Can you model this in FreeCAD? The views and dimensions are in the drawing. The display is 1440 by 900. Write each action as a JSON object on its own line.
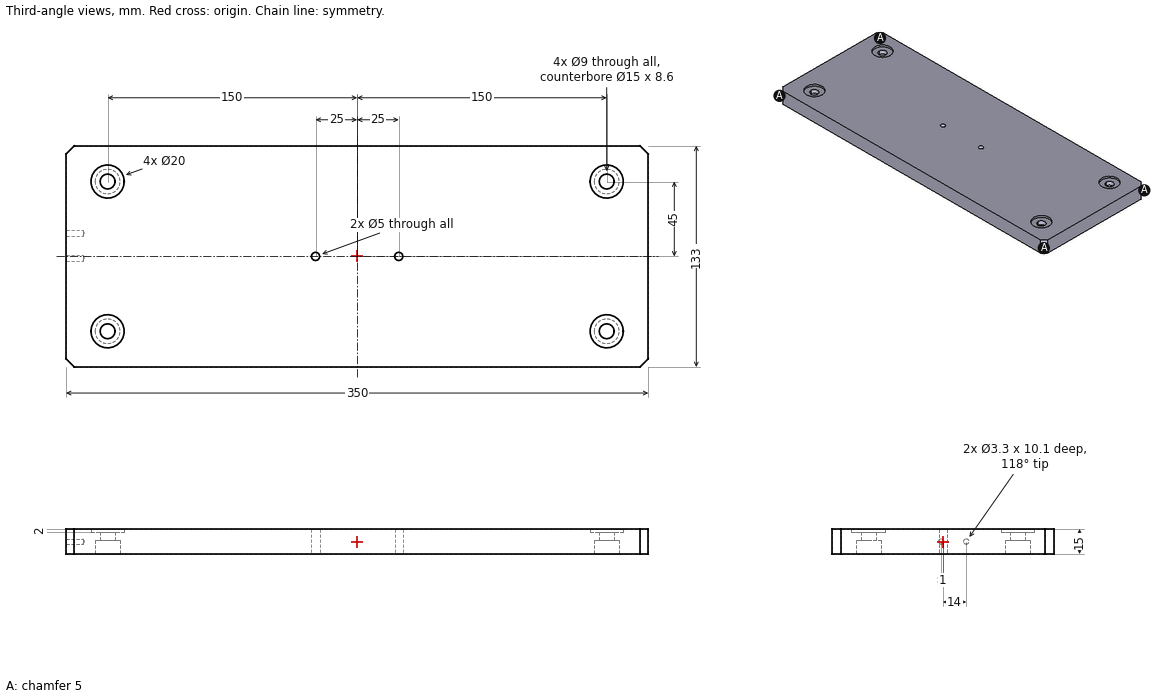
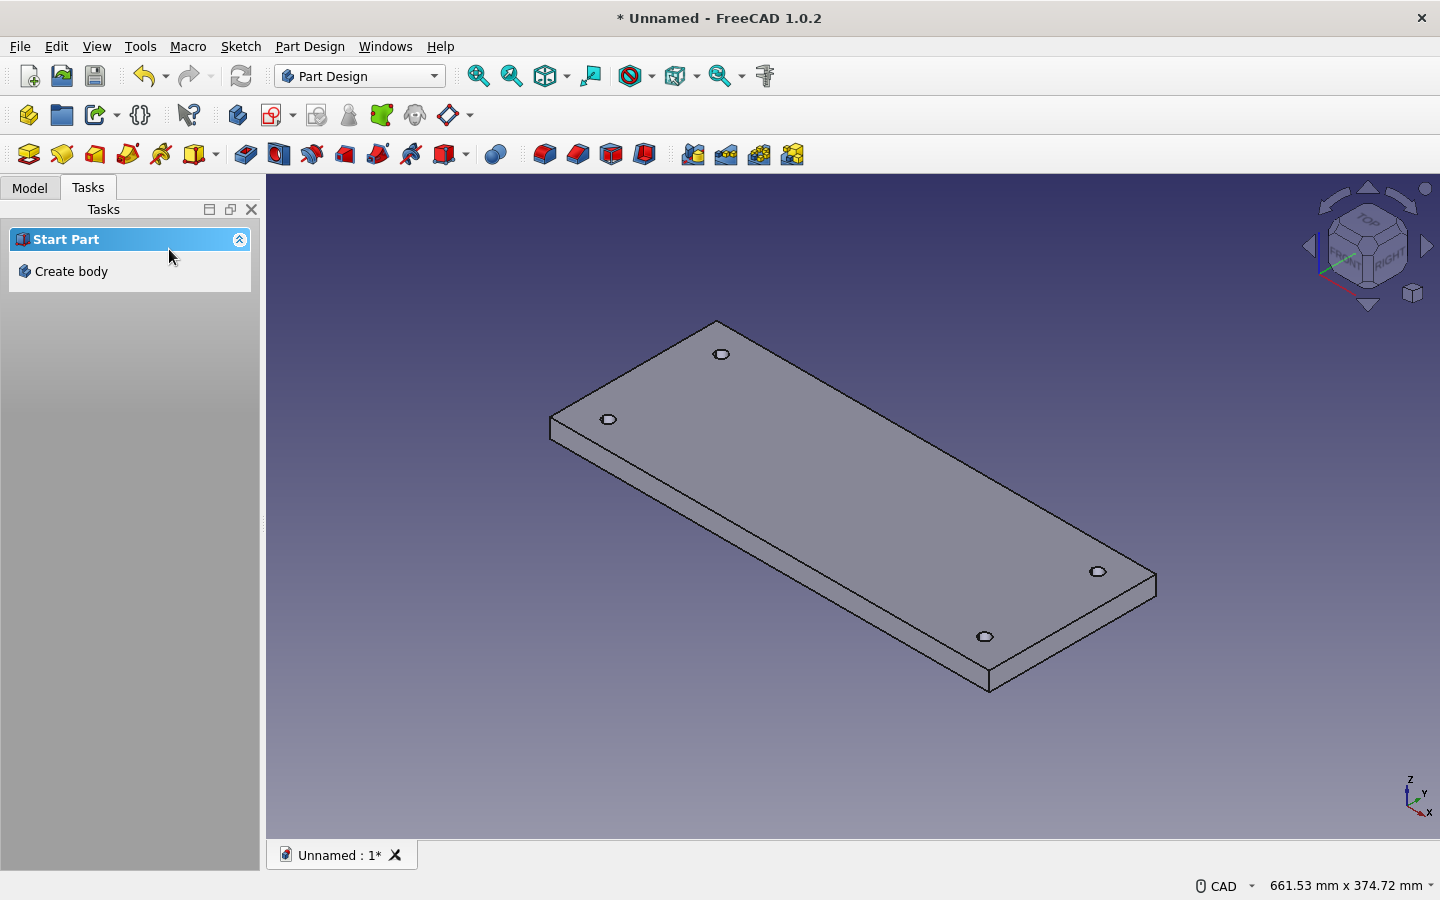
{"action": "left_click", "coordinate": [916, 531]}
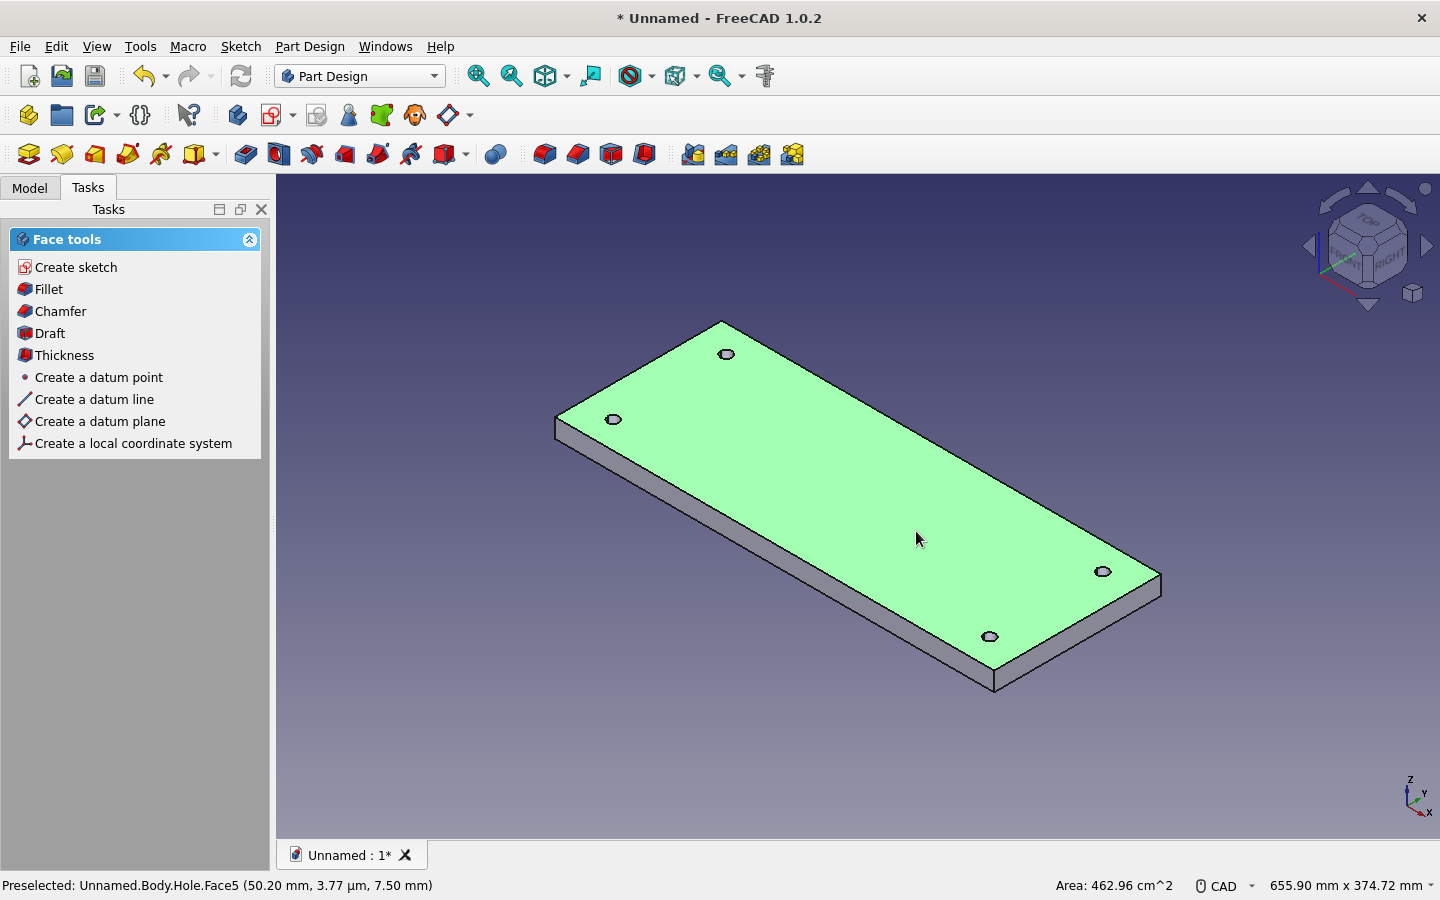
{"action": "left_click", "coordinate": [270, 116]}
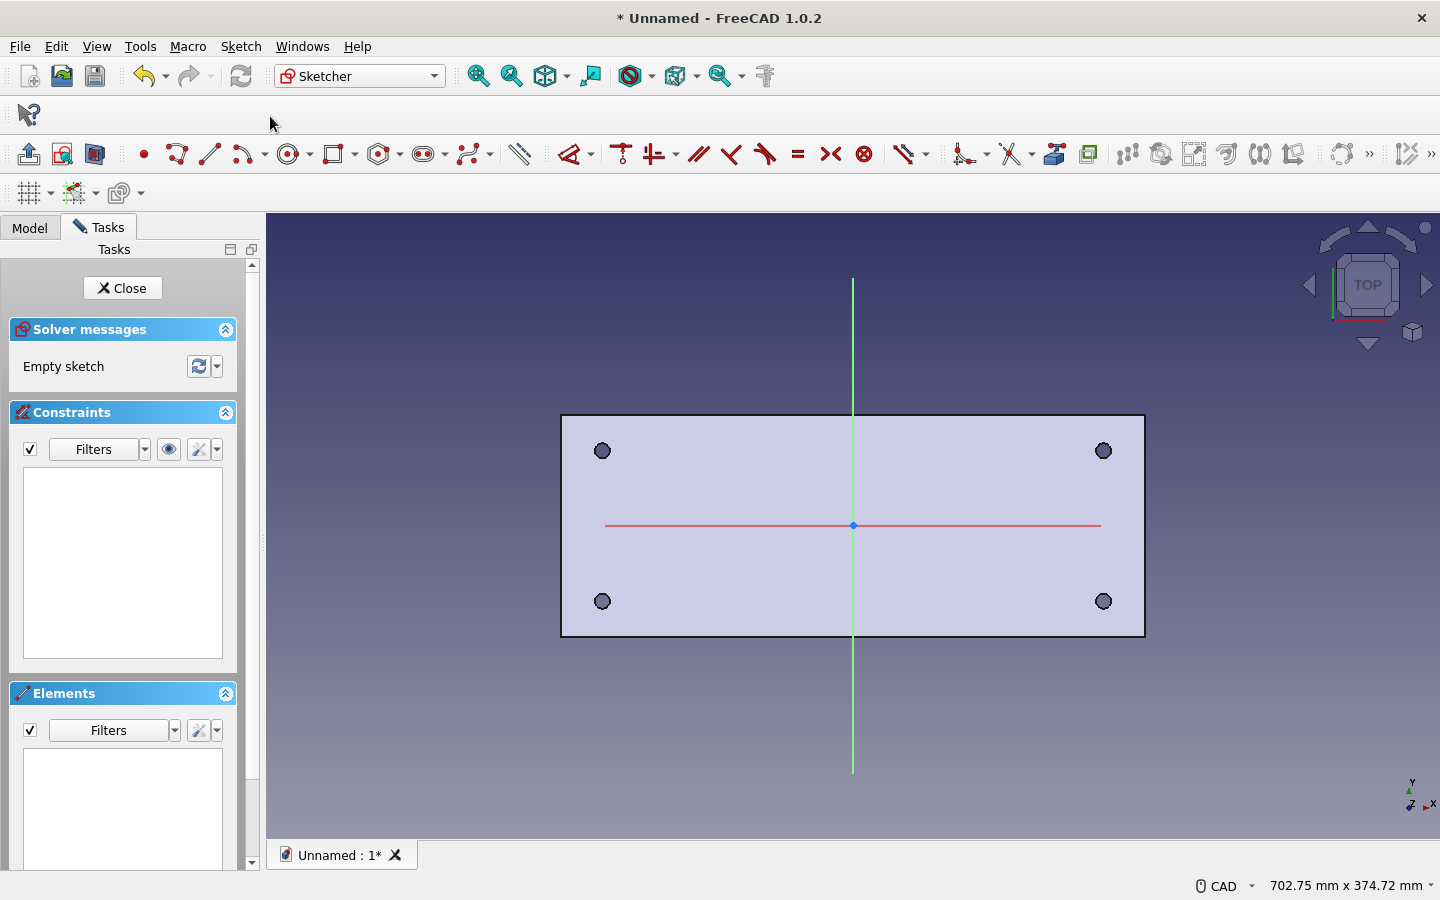
{"action": "scroll", "coordinate": [864, 526], "scroll_direction": "up", "scroll_amount": 10}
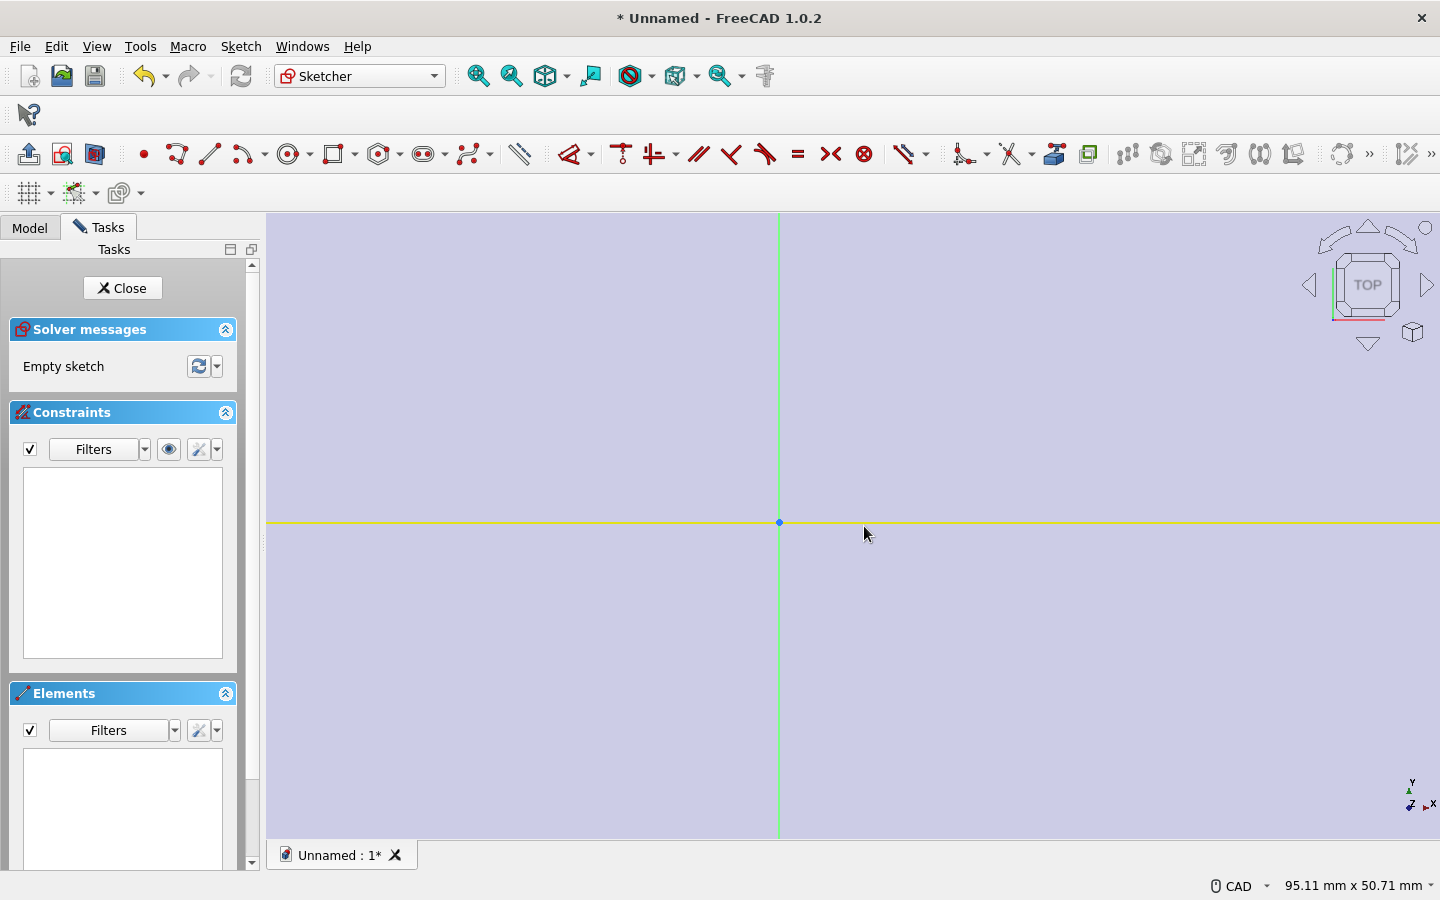
{"action": "key", "text": "g c"}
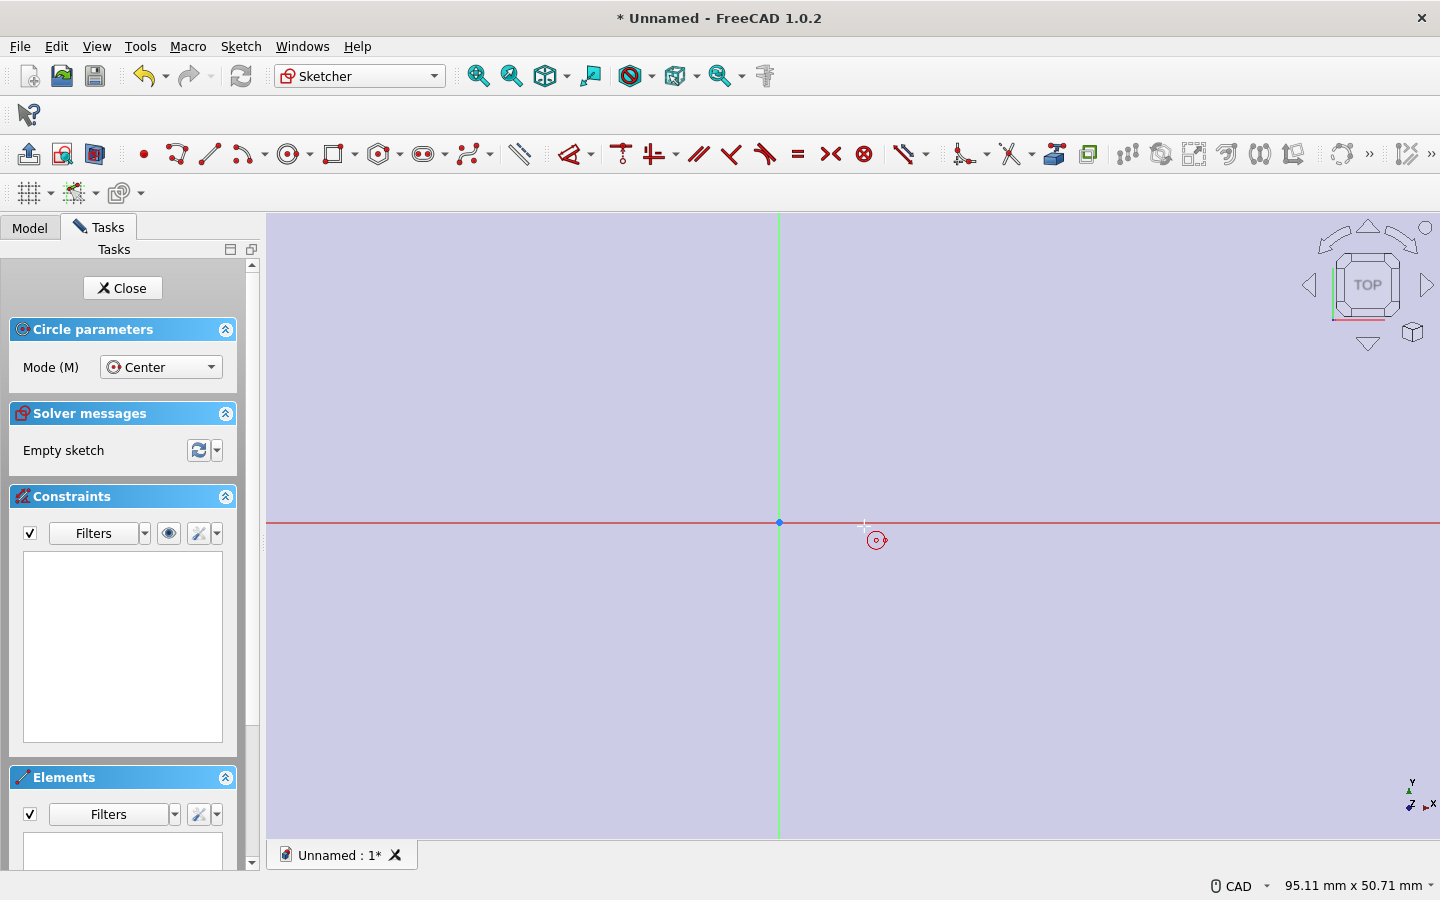
{"action": "left_click", "coordinate": [471, 523]}
{"action": "mouse_move", "coordinate": [493, 501]}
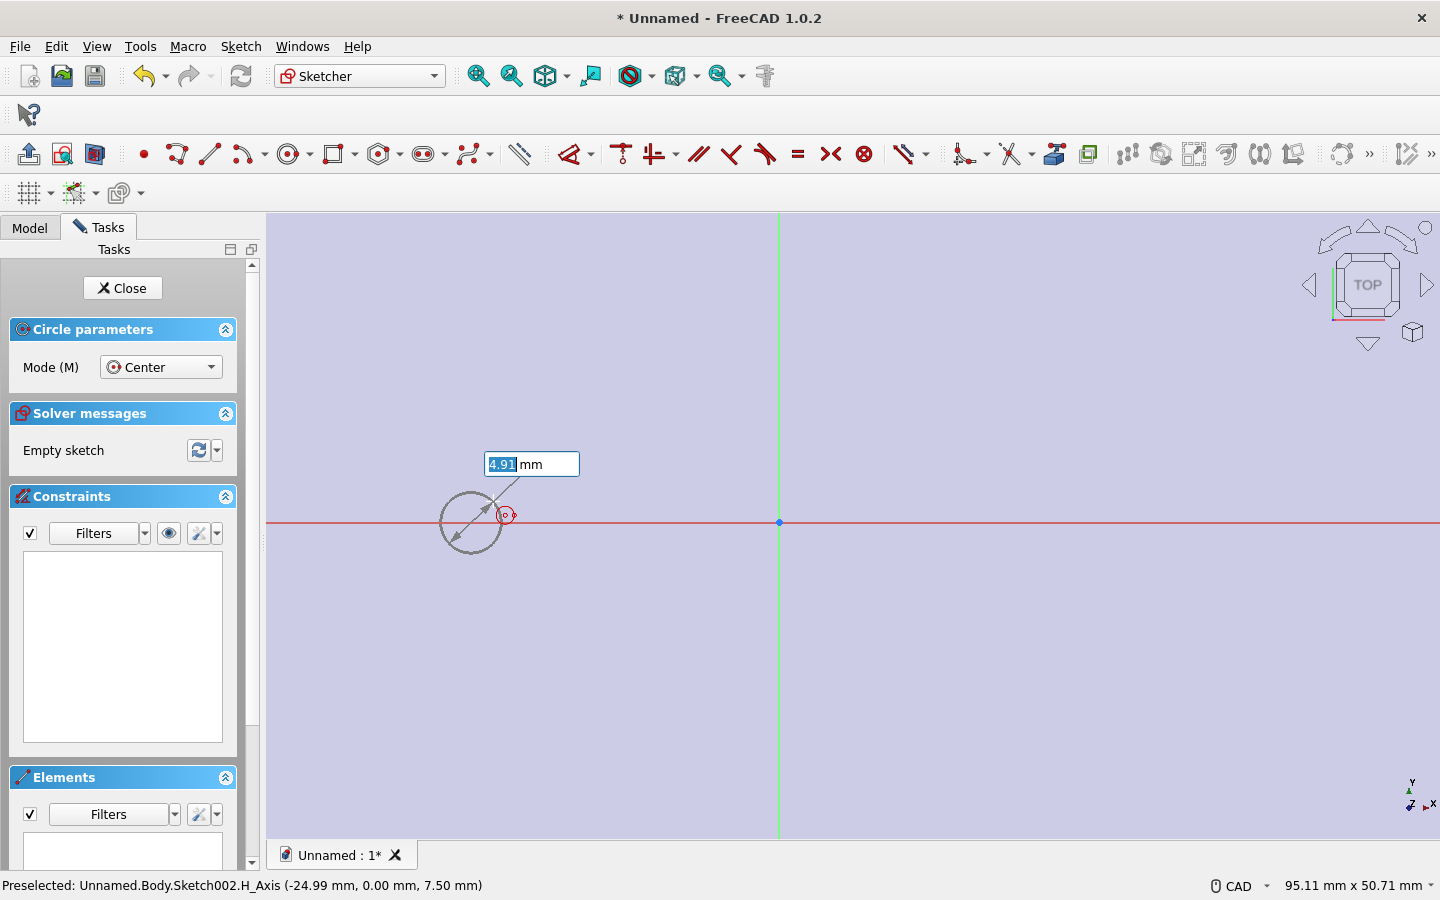
{"action": "type", "text": "5"}
{"action": "key", "text": "Return"}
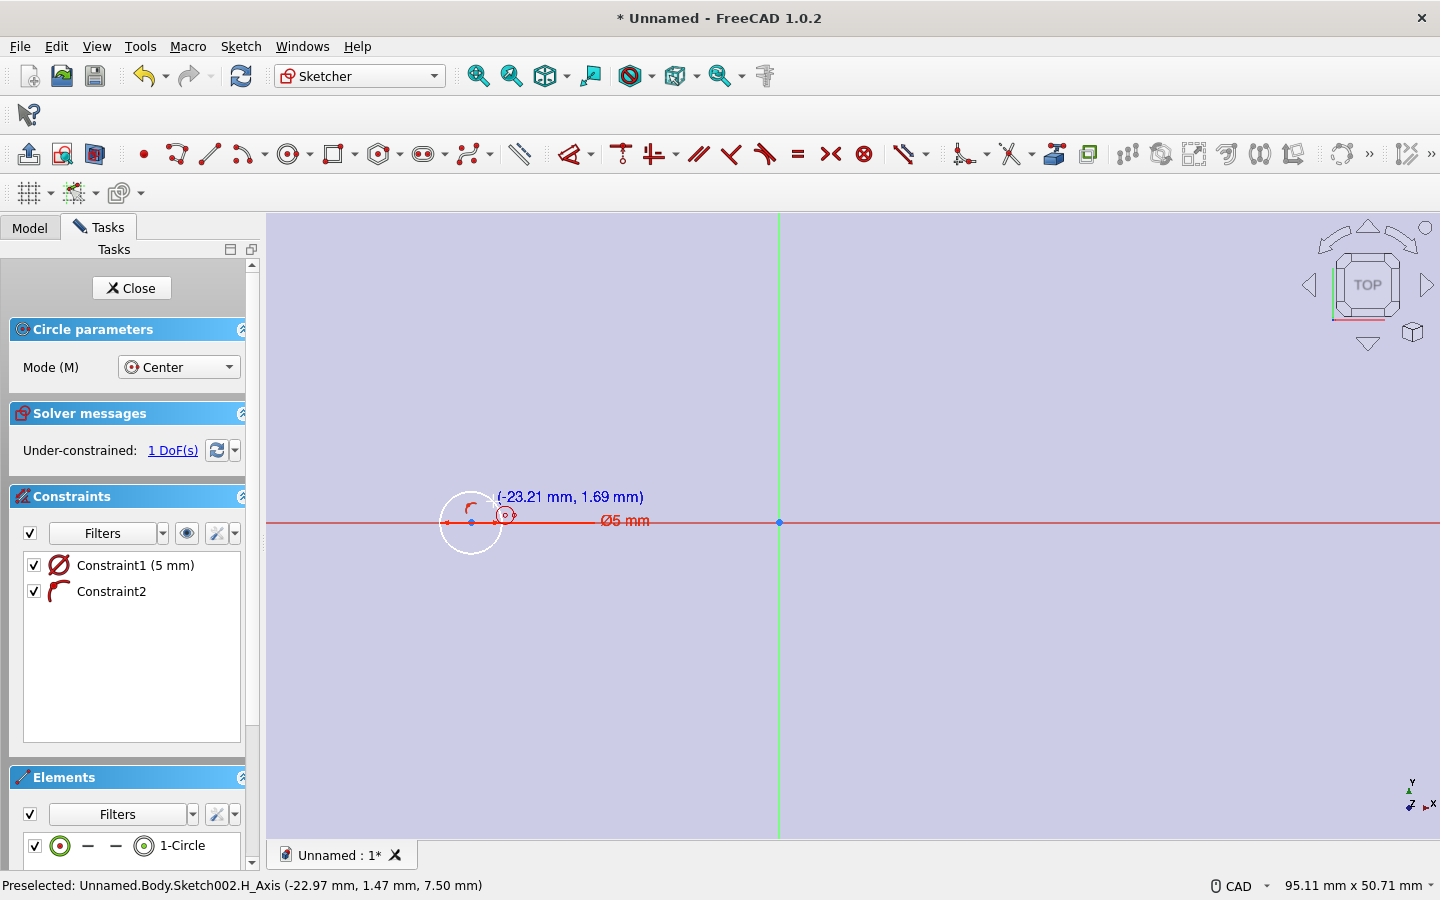
{"action": "left_click", "coordinate": [1088, 523]}
{"action": "mouse_move", "coordinate": [1110, 501]}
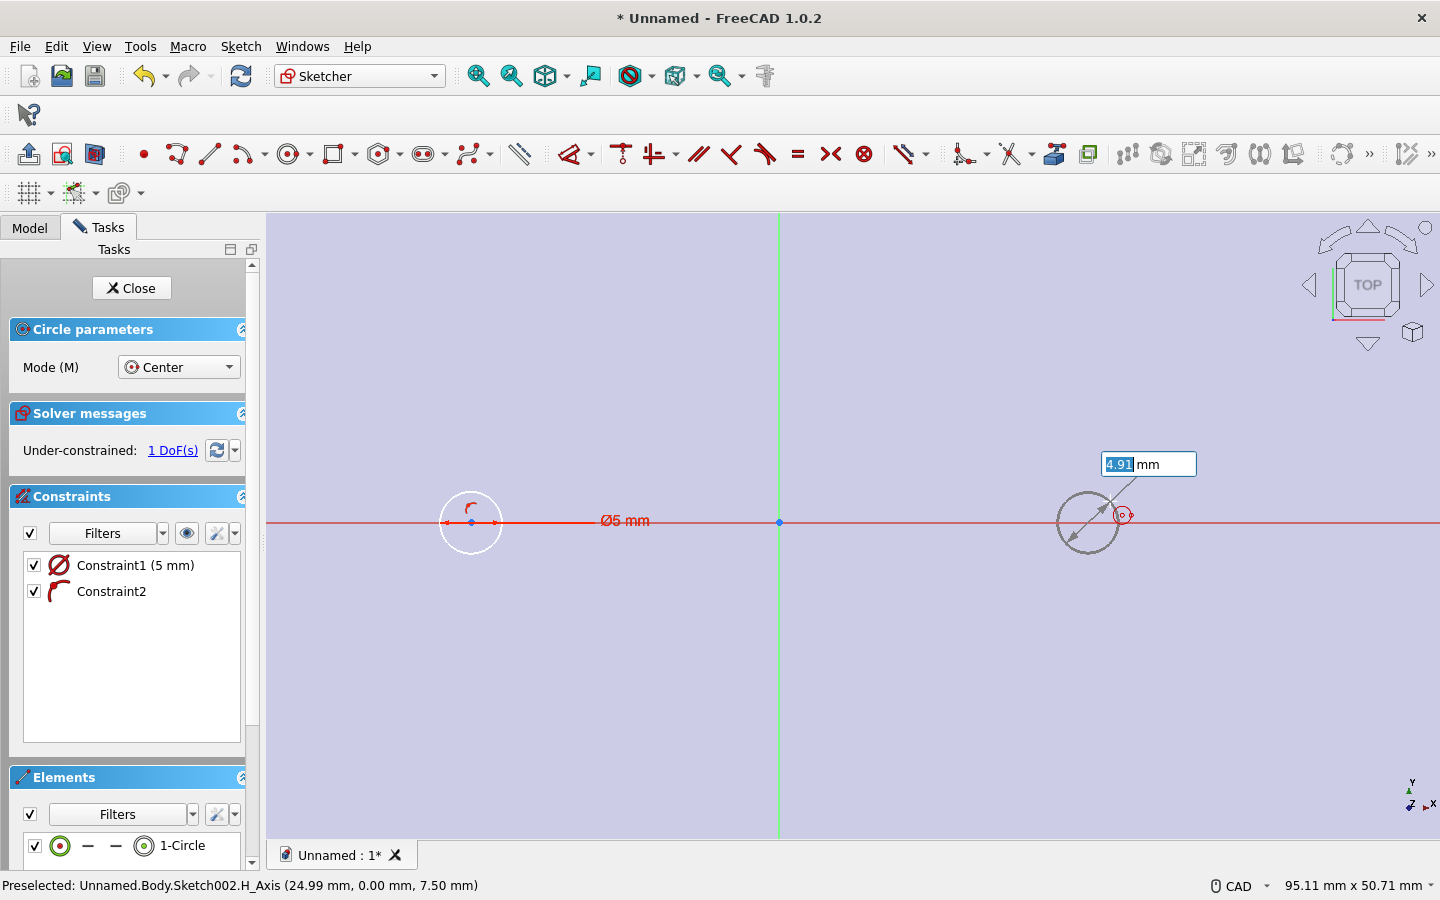
{"action": "type", "text": "5"}
{"action": "key", "text": "Return"}
{"action": "key", "text": "Escape"}